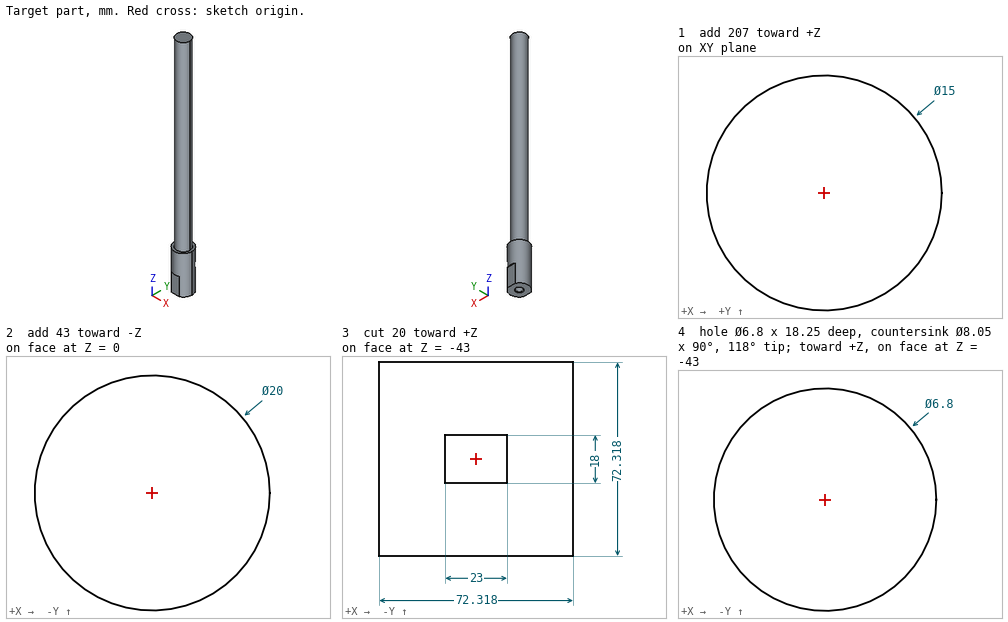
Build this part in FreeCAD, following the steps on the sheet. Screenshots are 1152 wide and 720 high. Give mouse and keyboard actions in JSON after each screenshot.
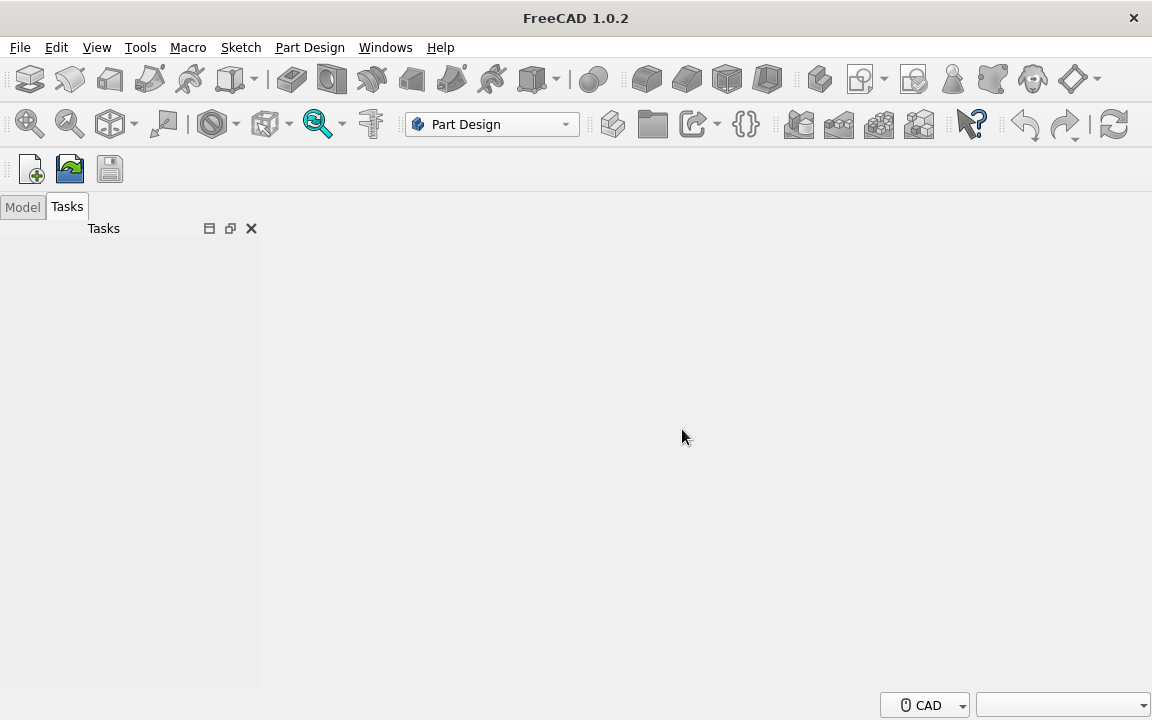
{"action": "key", "text": "ctrl+n"}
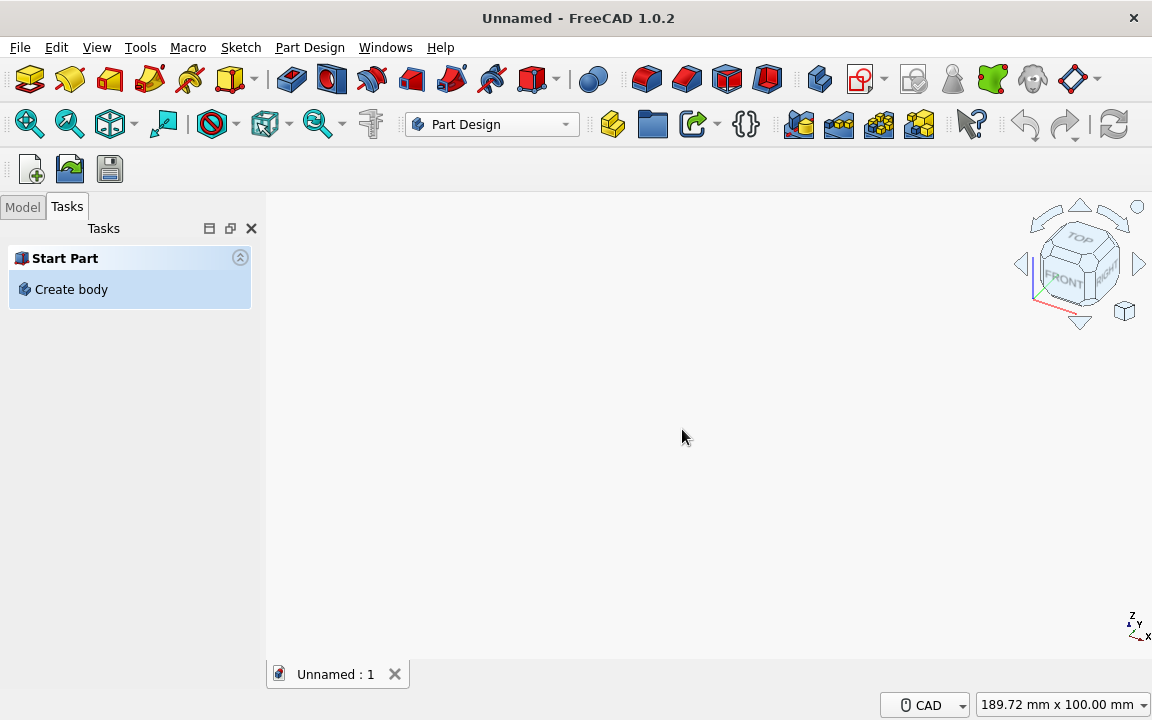
{"action": "left_click", "coordinate": [860, 80]}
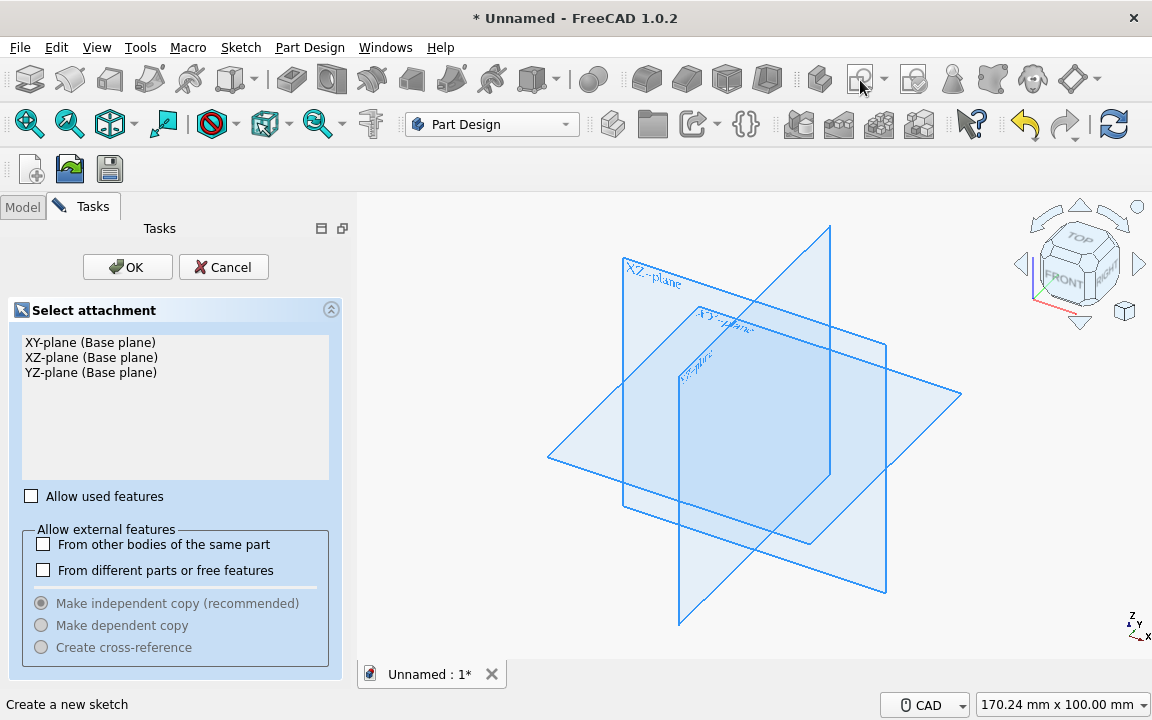
{"action": "left_click", "coordinate": [82, 342]}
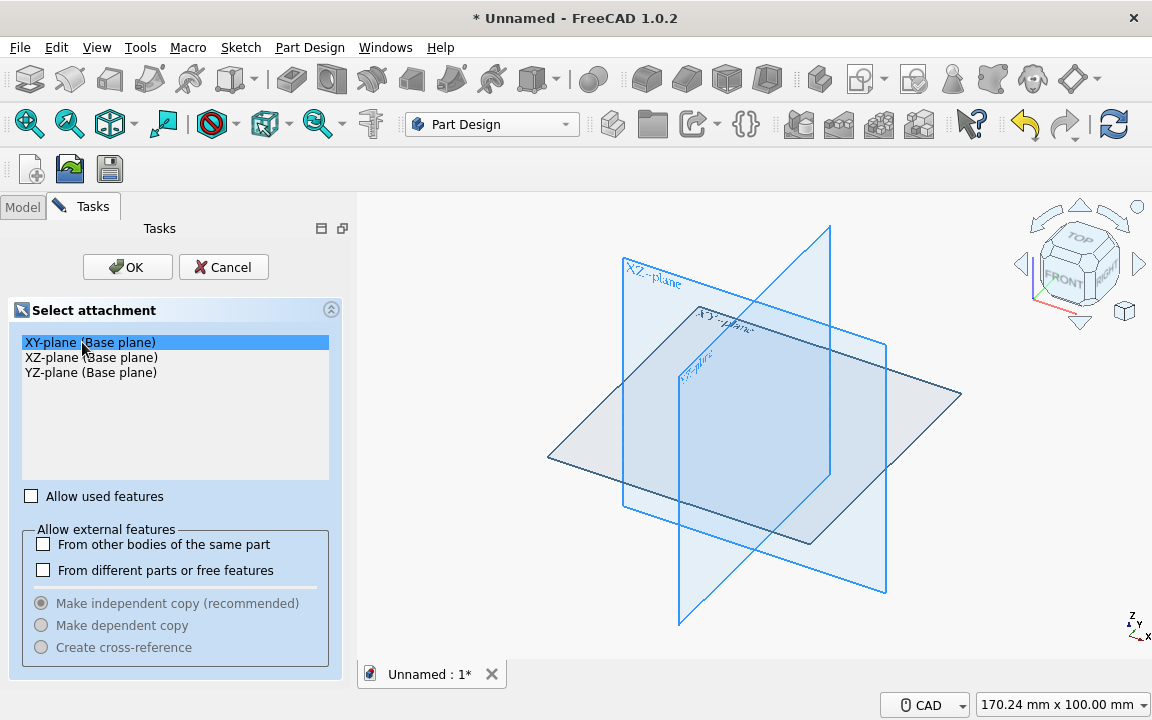
{"action": "left_click", "coordinate": [128, 267]}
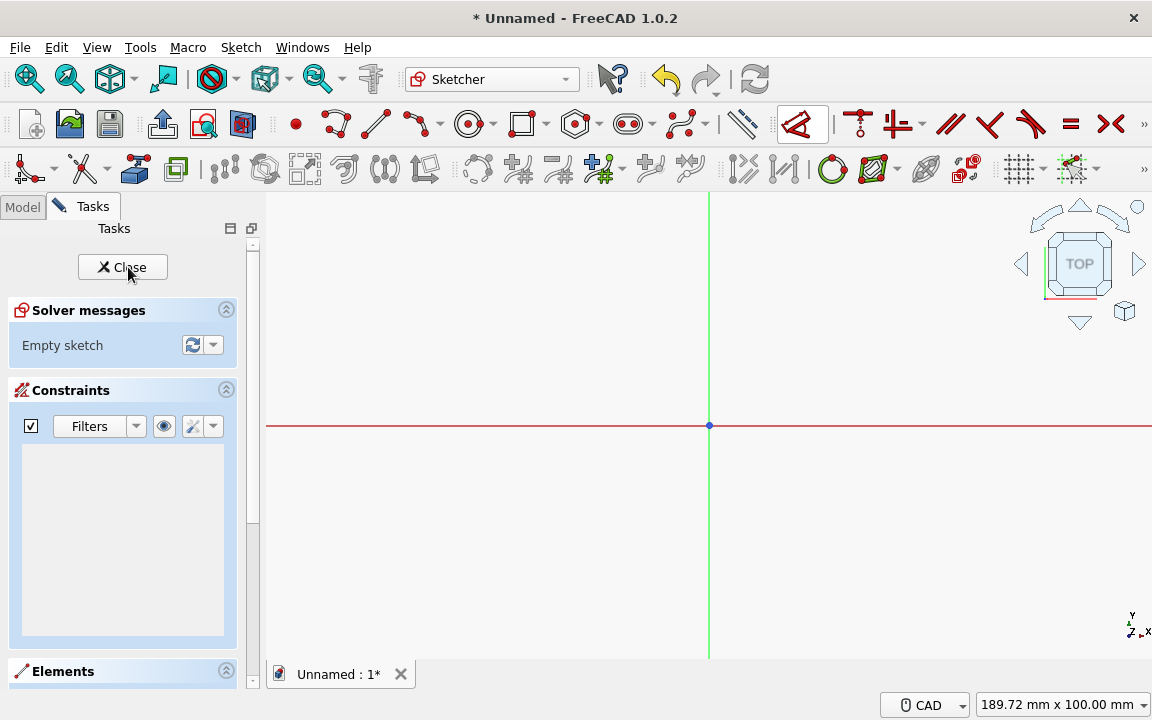
{"action": "scroll", "coordinate": [731, 426], "scroll_direction": "up", "scroll_amount": 7}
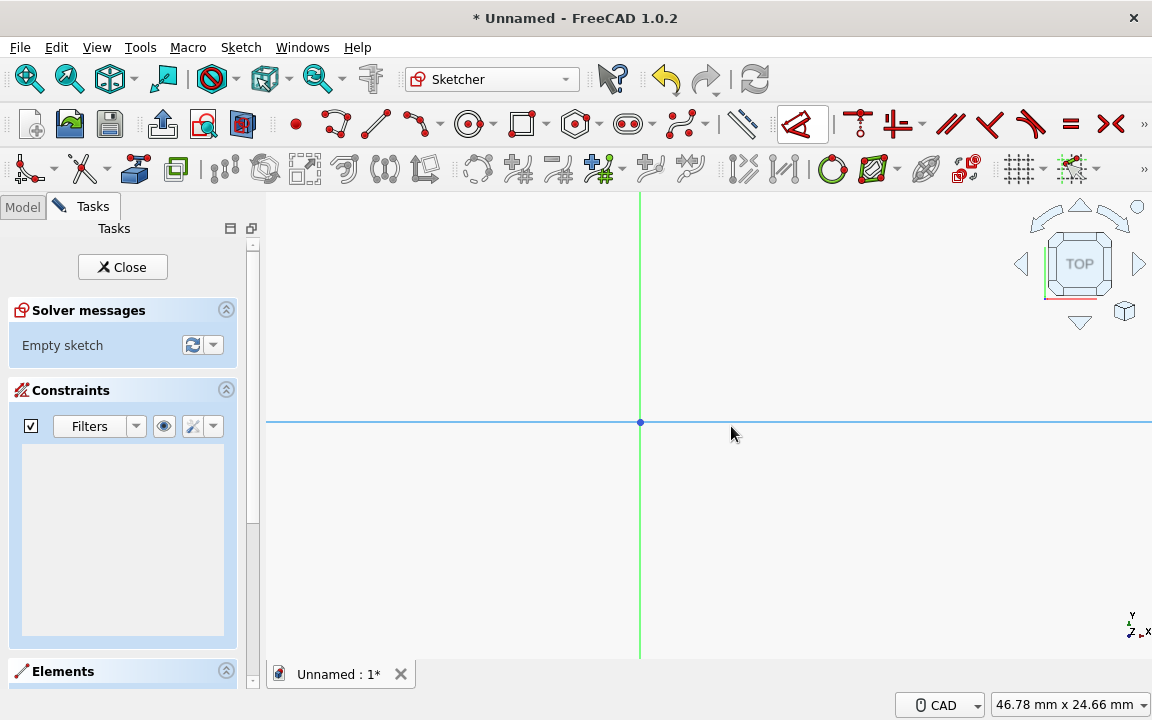
{"action": "key", "text": "g c"}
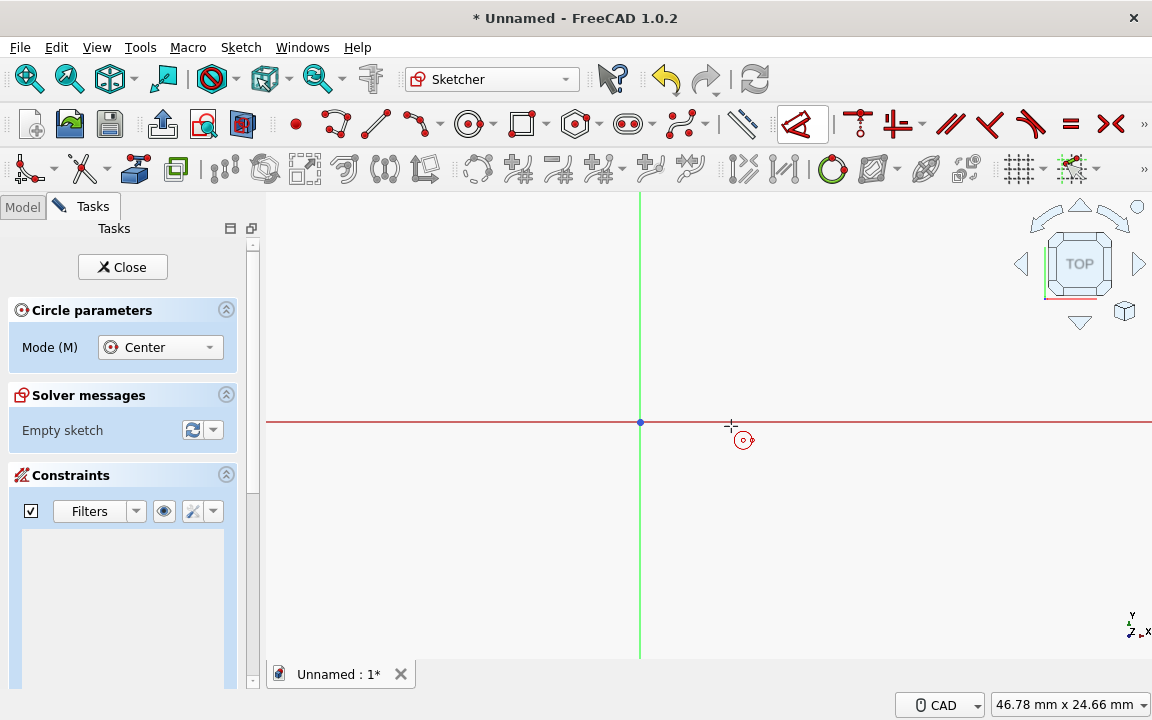
{"action": "left_click", "coordinate": [640, 422]}
{"action": "mouse_move", "coordinate": [741, 322]}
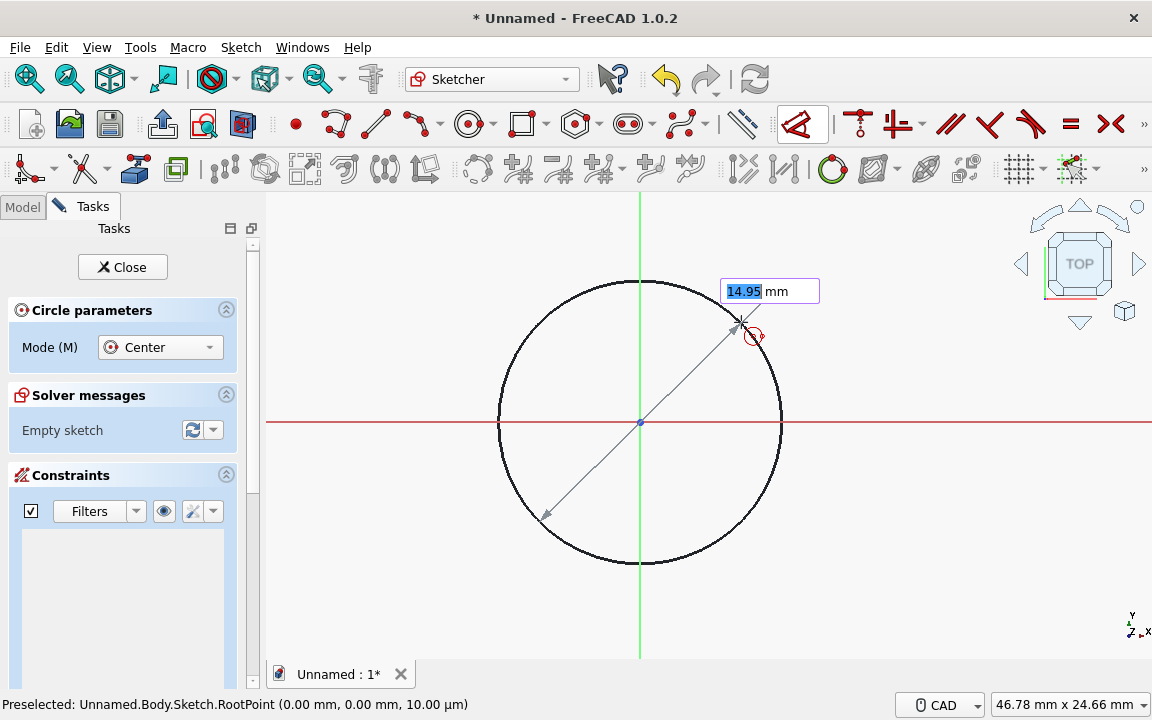
{"action": "type", "text": "15"}
{"action": "key", "text": "Return"}
{"action": "key", "text": "Escape"}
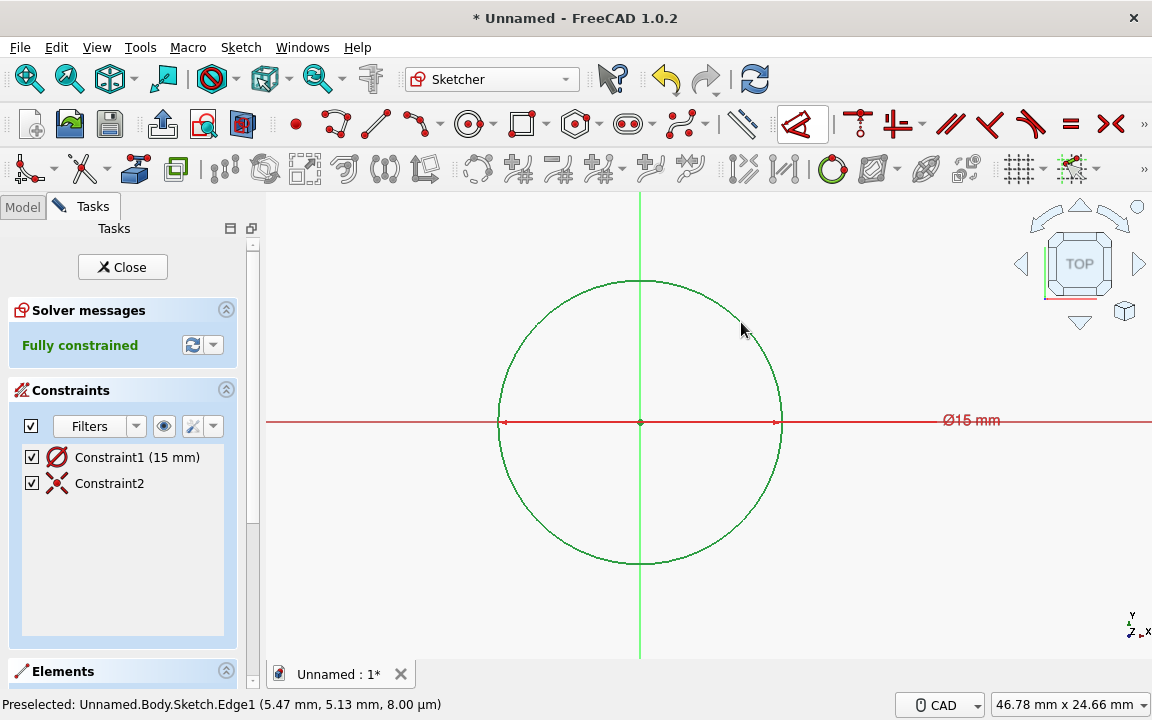
{"action": "left_click", "coordinate": [123, 267]}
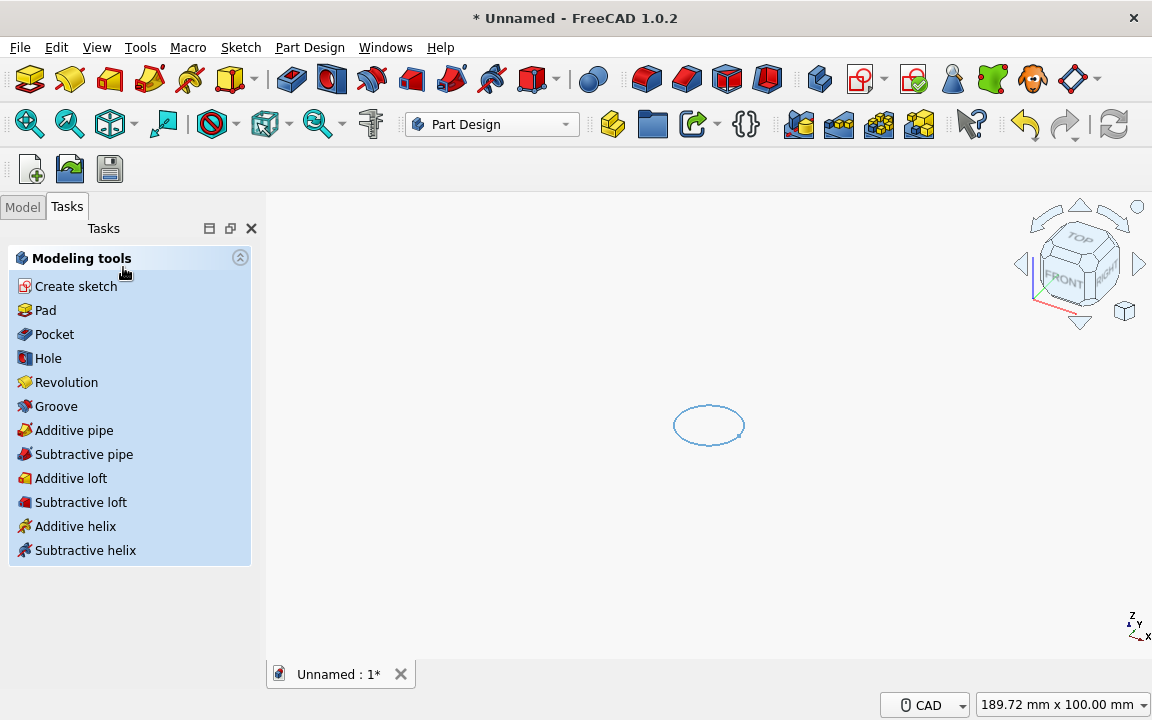
{"action": "left_click", "coordinate": [30, 80]}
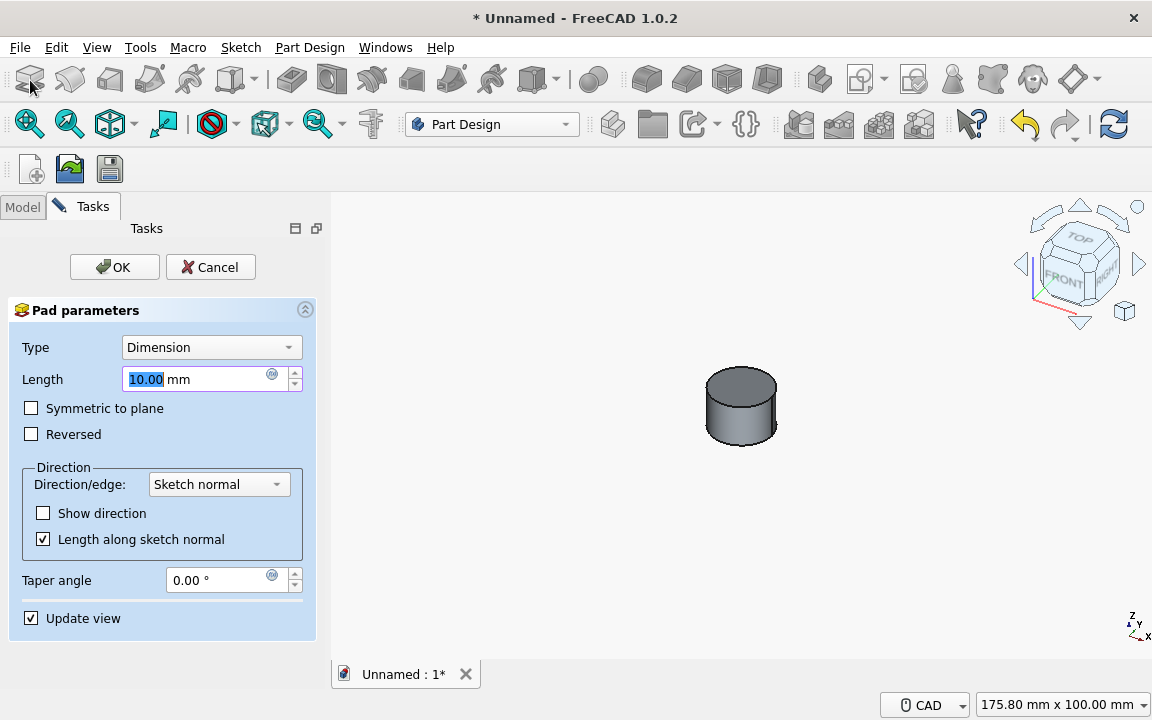
{"action": "type", "text": "207"}
{"action": "key", "text": "Tab"}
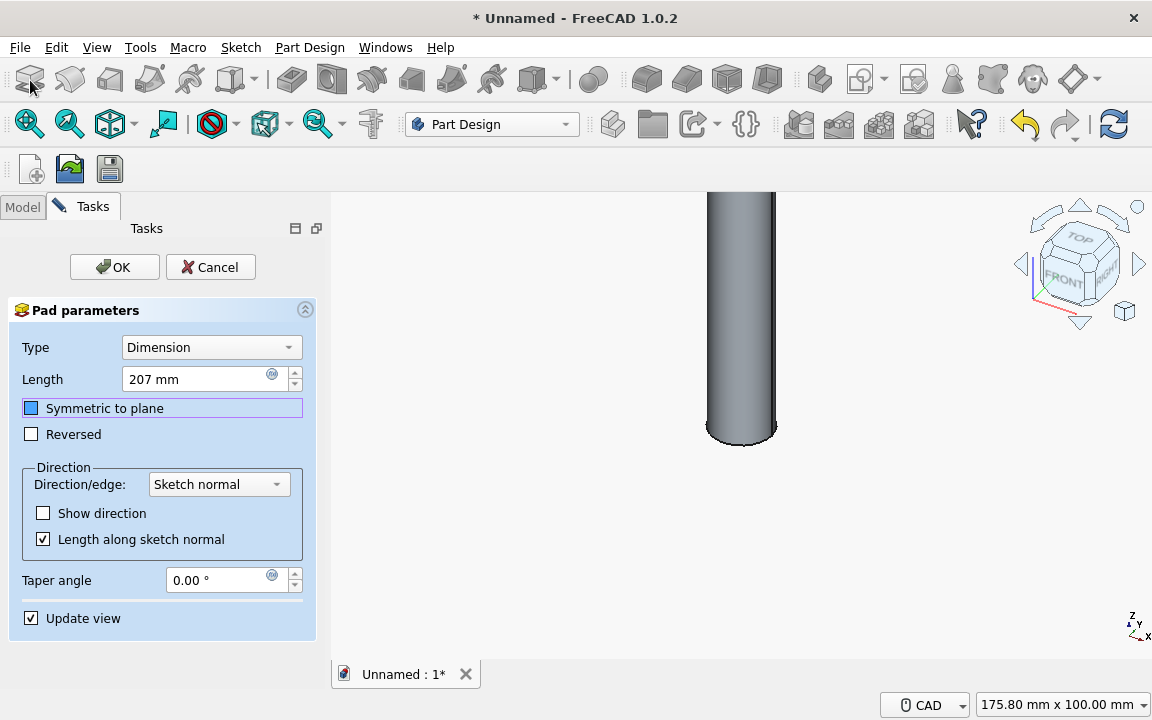
{"action": "left_click", "coordinate": [115, 267]}